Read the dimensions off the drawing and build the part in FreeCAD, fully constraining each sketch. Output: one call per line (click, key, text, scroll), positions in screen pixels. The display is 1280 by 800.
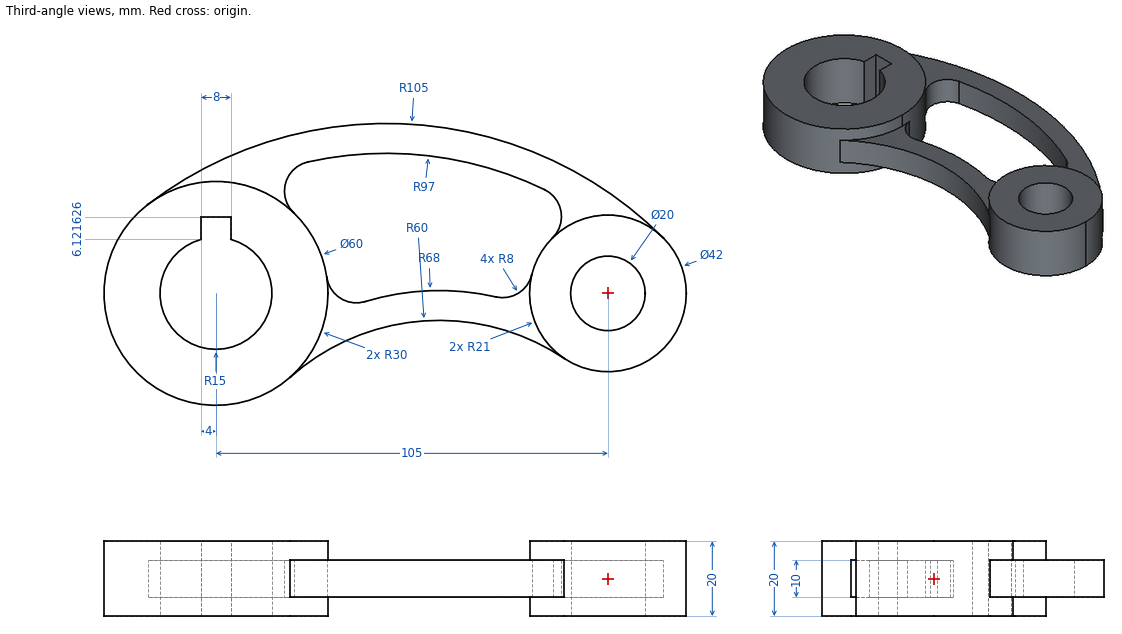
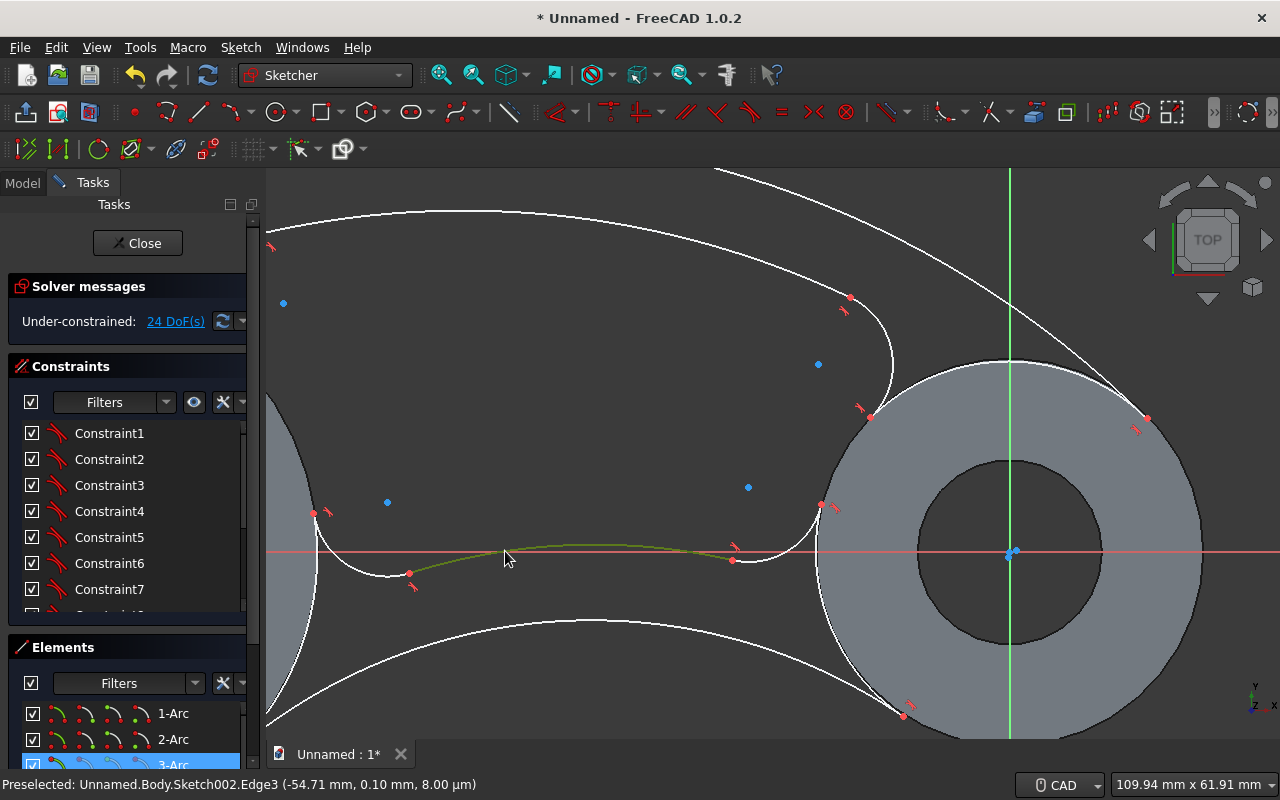
click(703, 631)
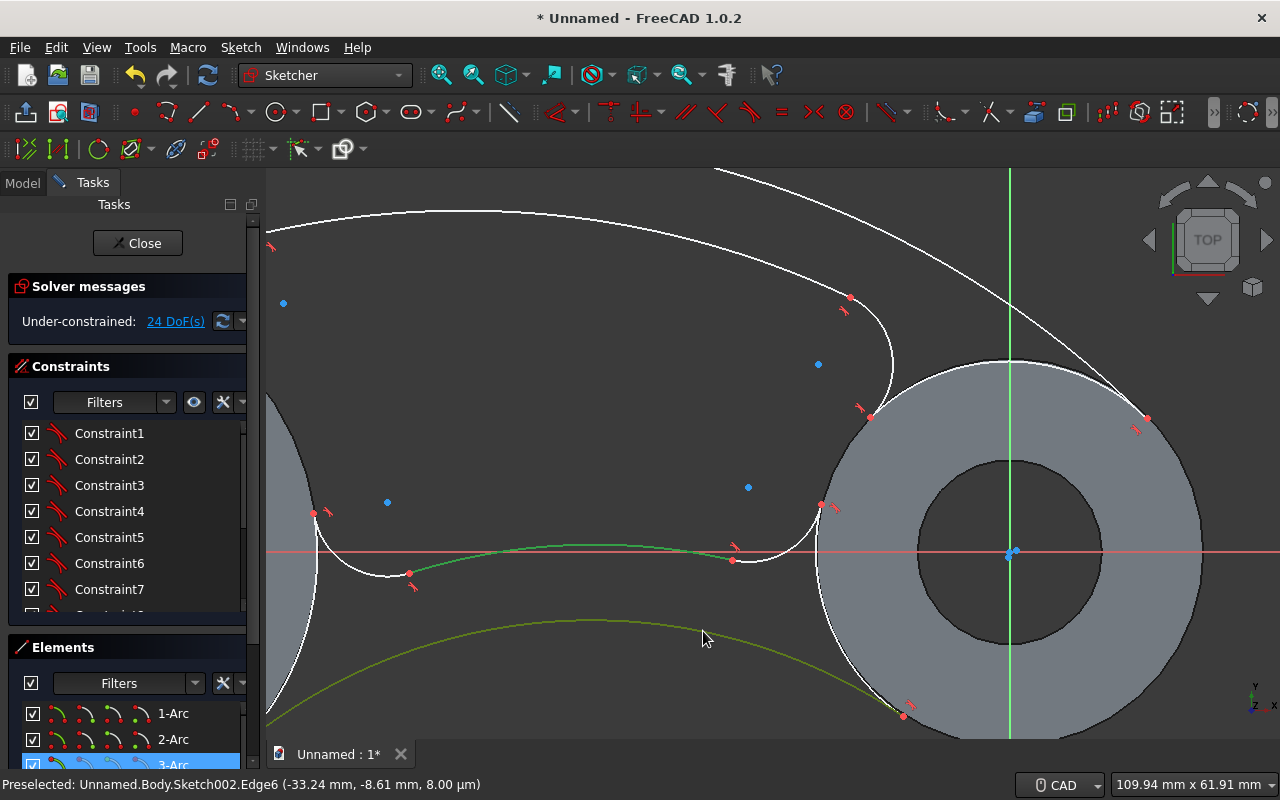
key(c)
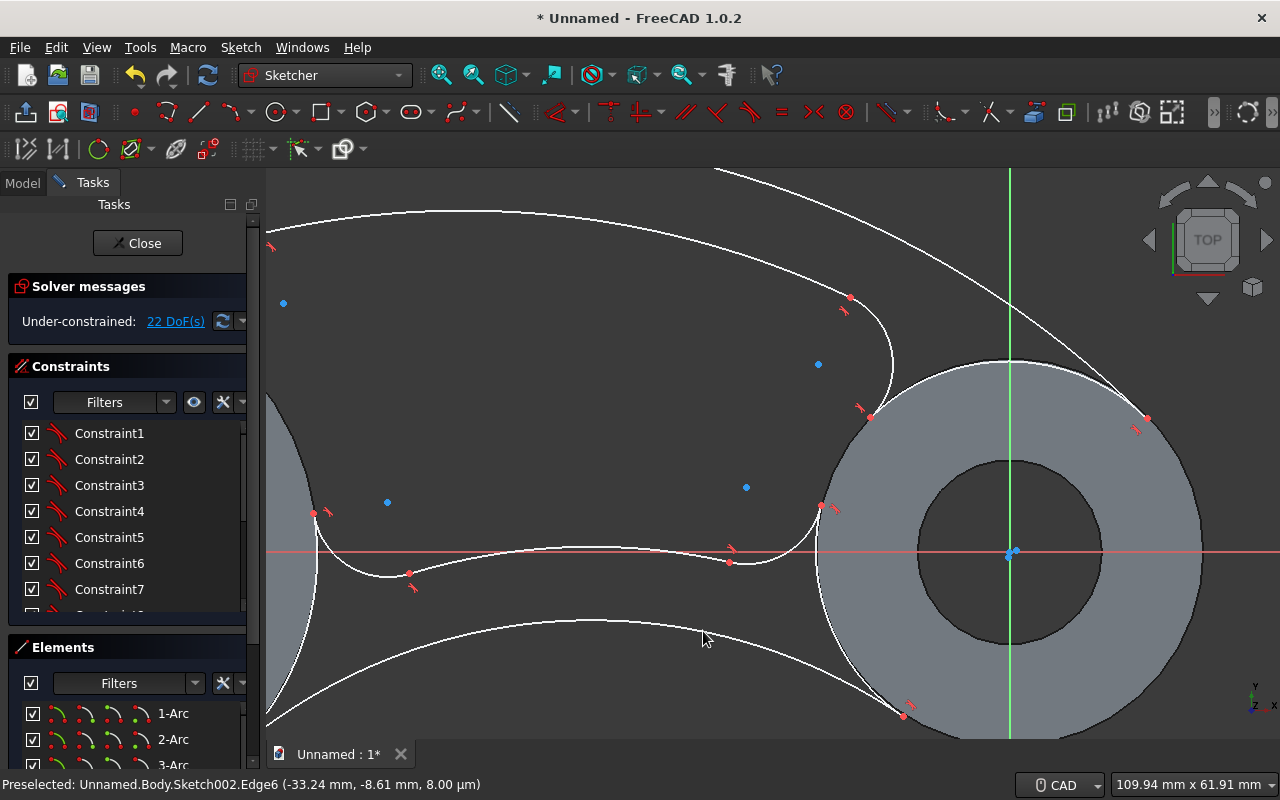
click(314, 595)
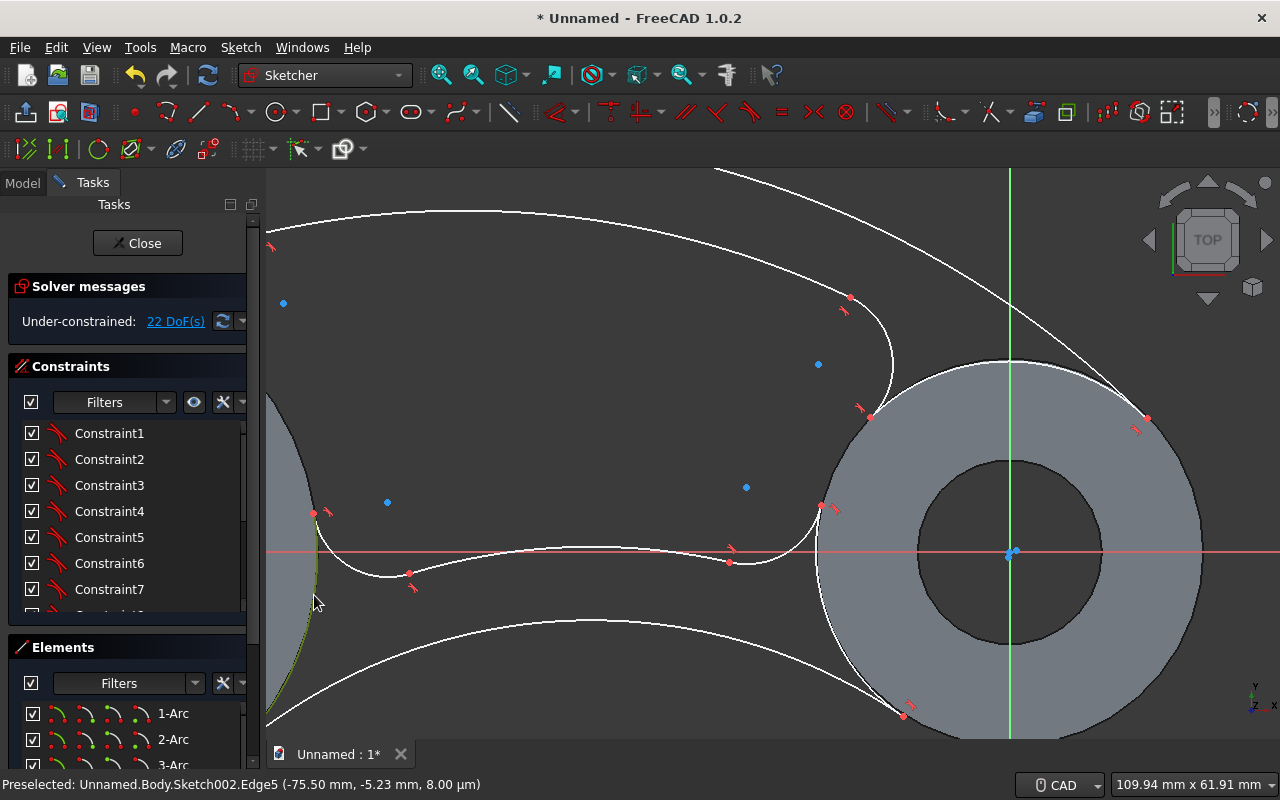
scroll(864, 459, down, 4)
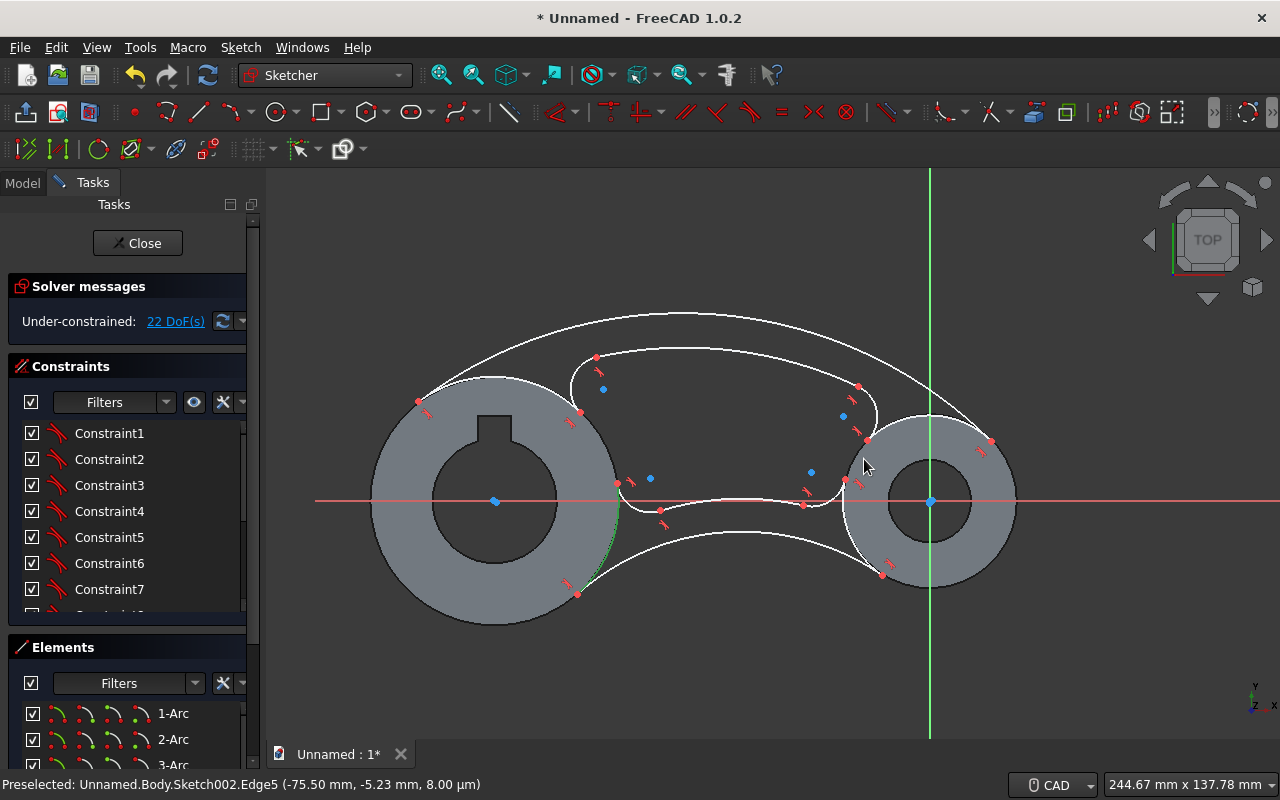
click(536, 384)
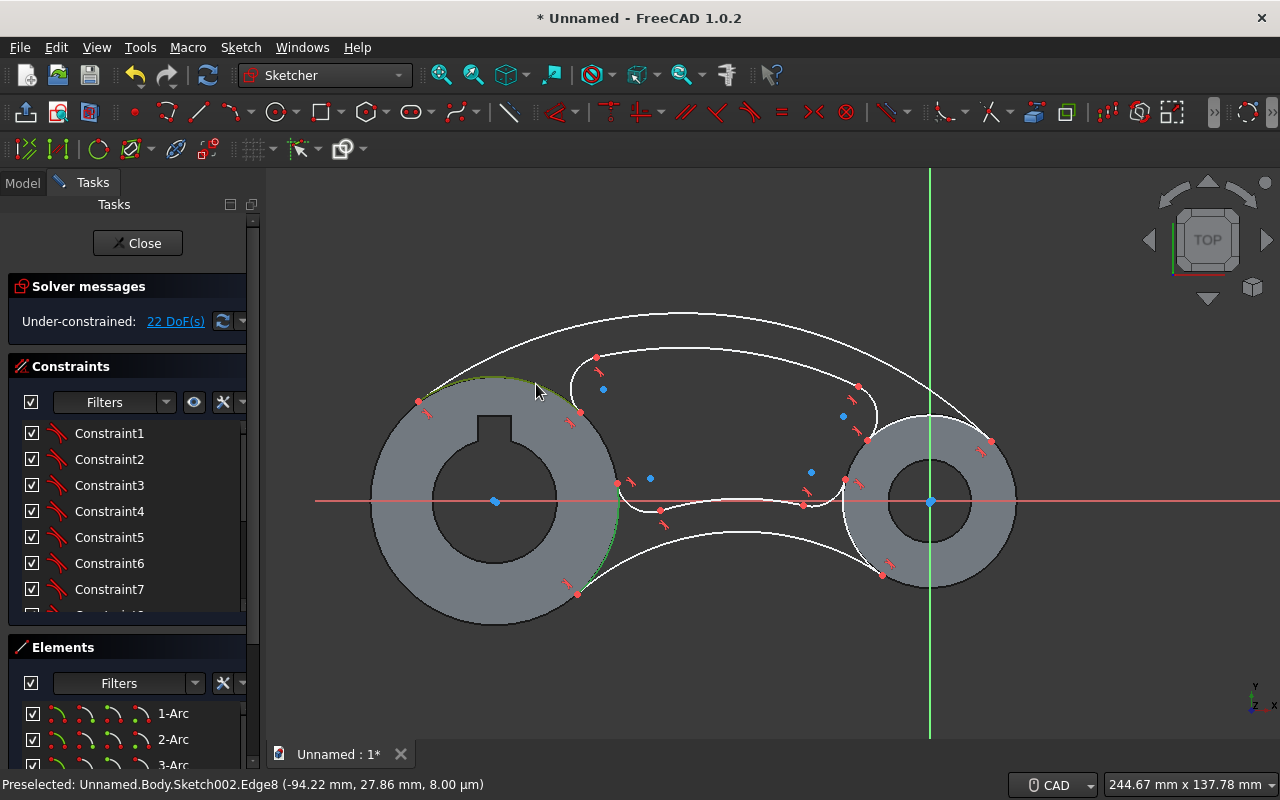
key(c)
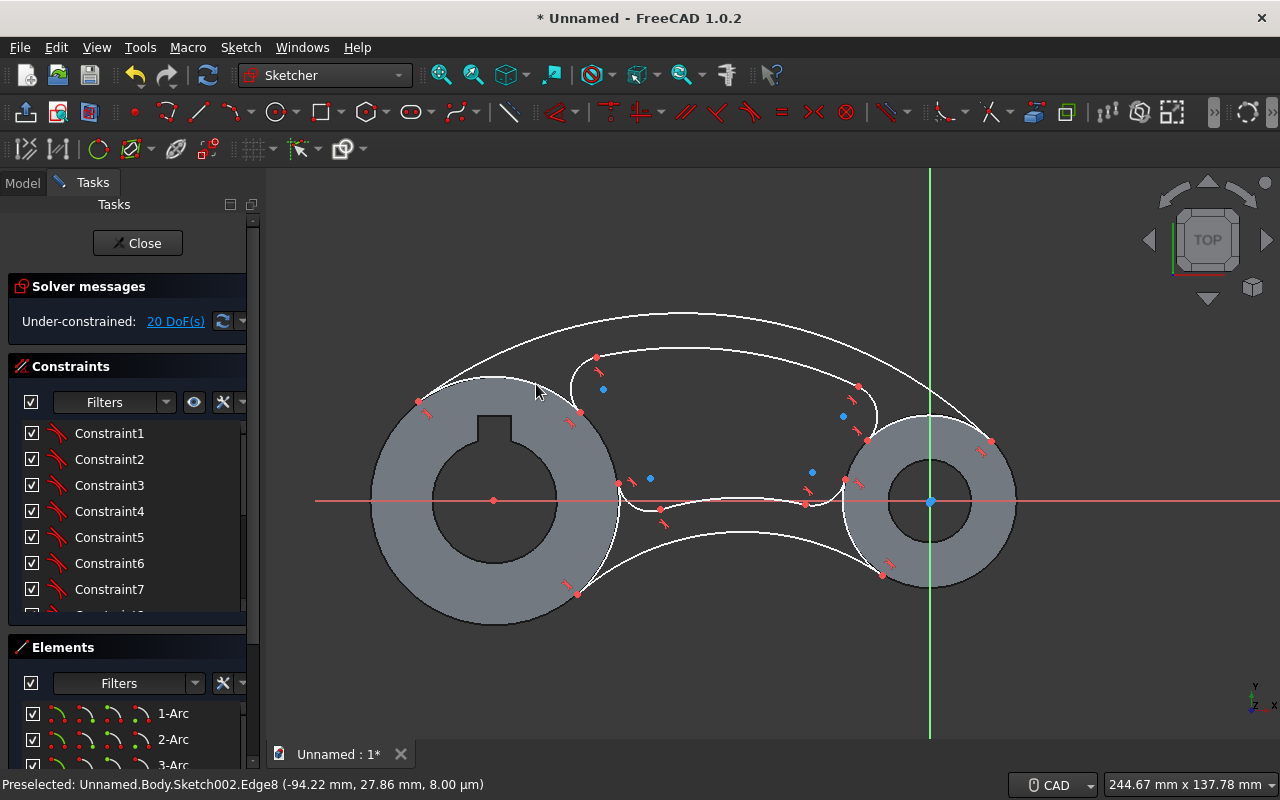
click(835, 341)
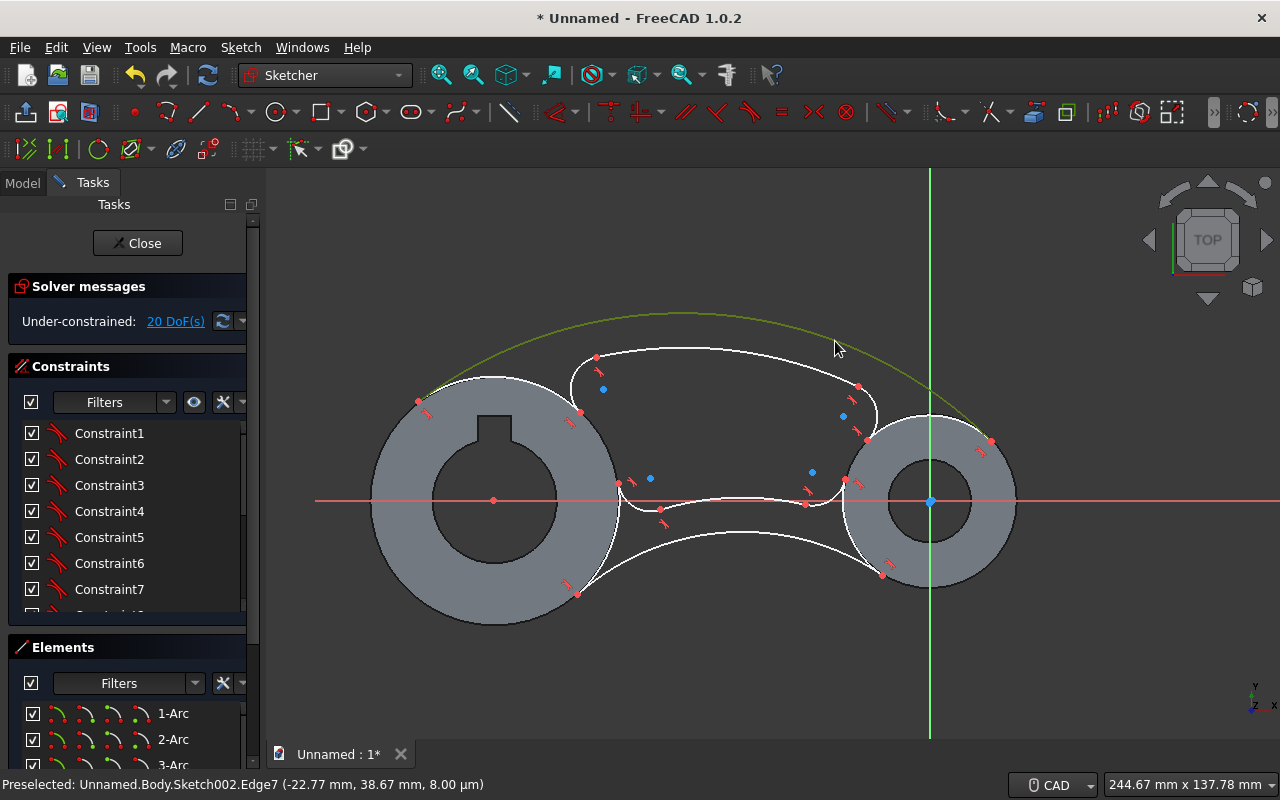
click(783, 360)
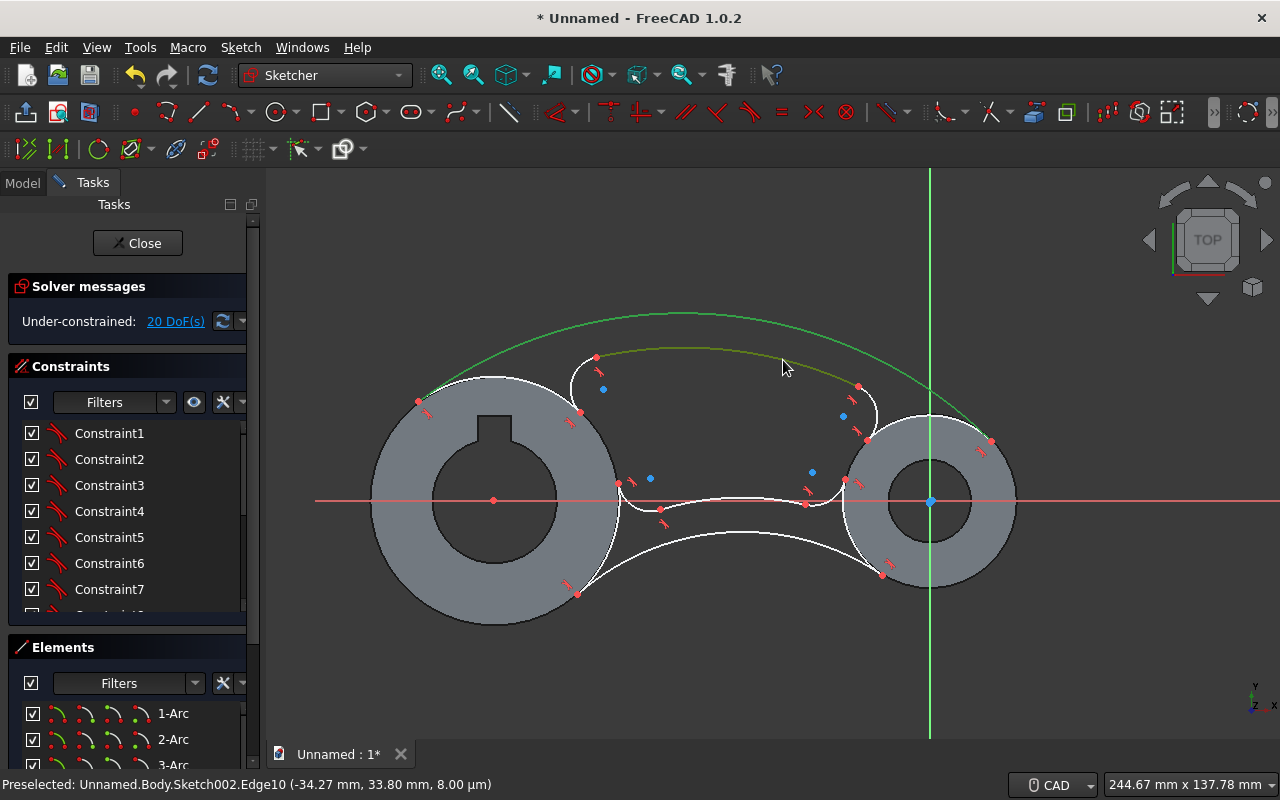
click(610, 112)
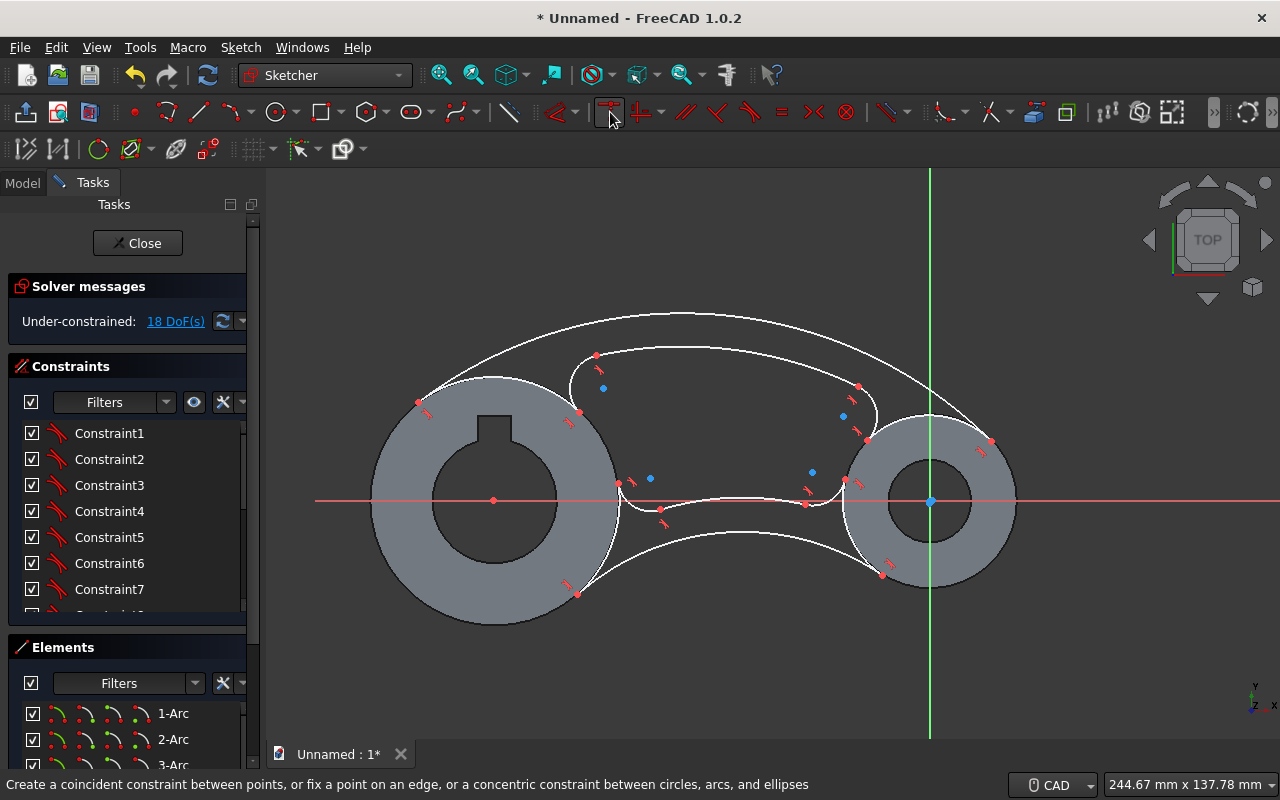
scroll(843, 512, up, 2)